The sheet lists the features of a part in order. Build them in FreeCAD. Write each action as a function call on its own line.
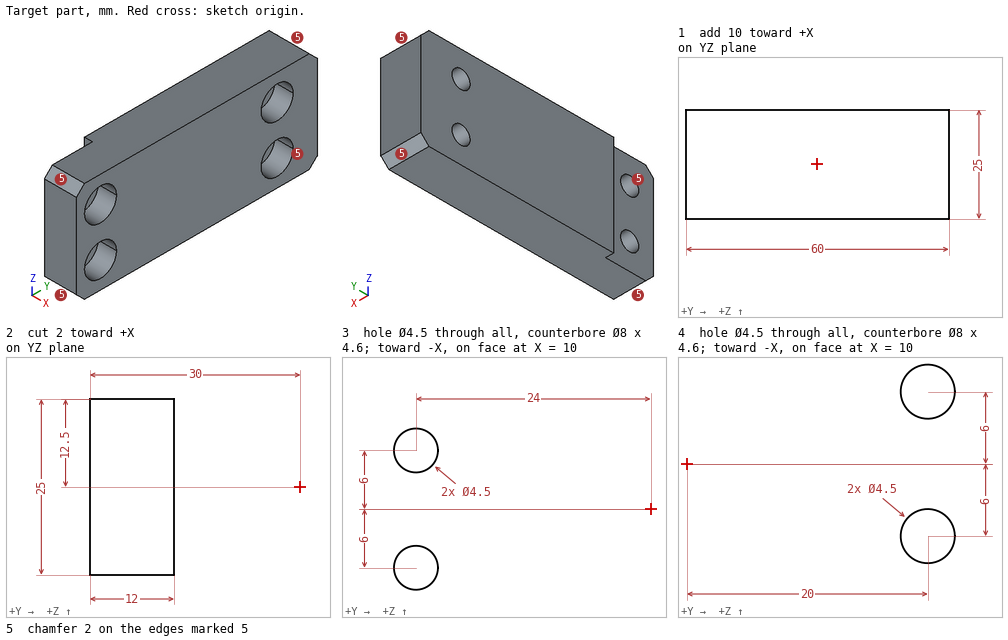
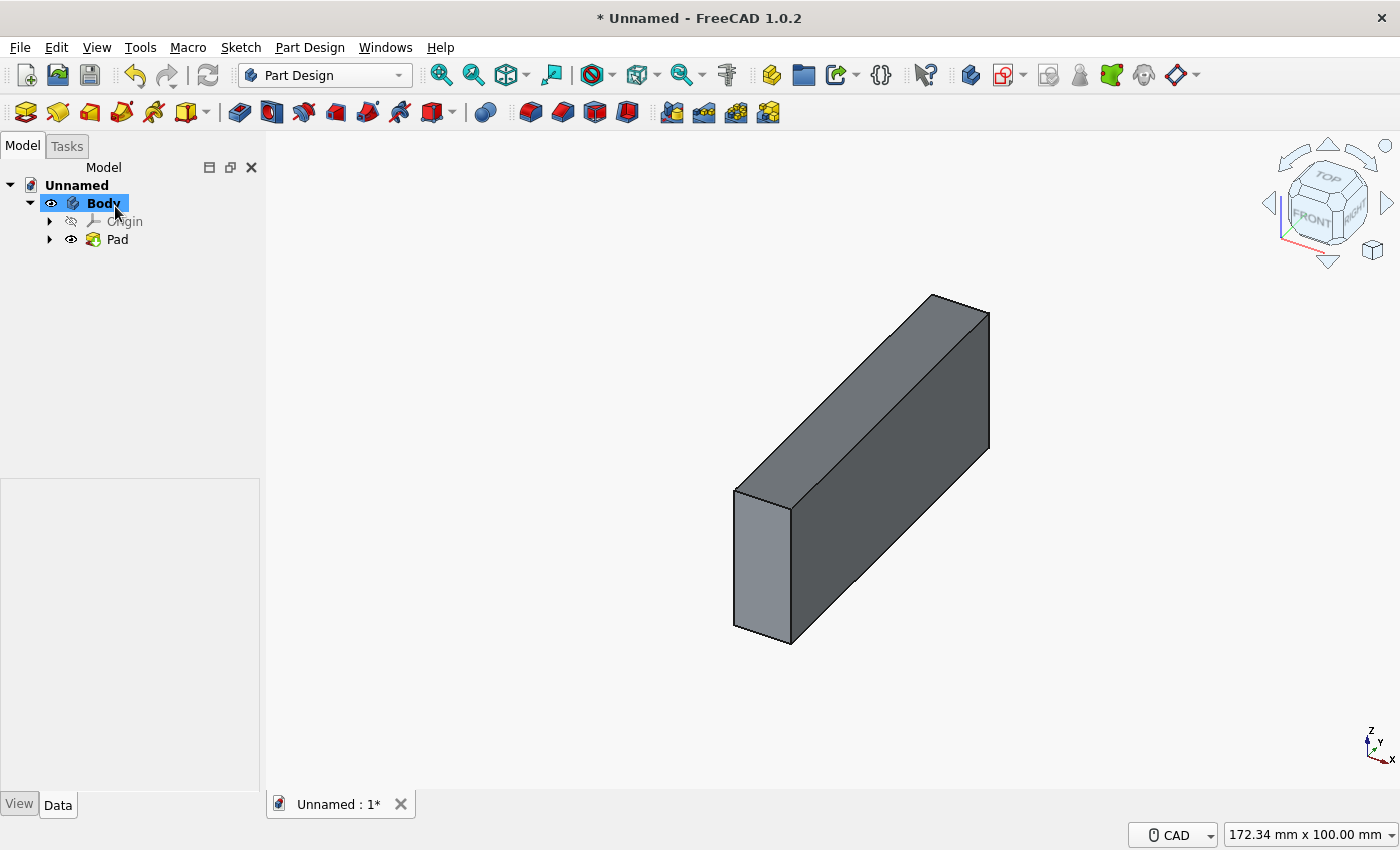
click(1004, 76)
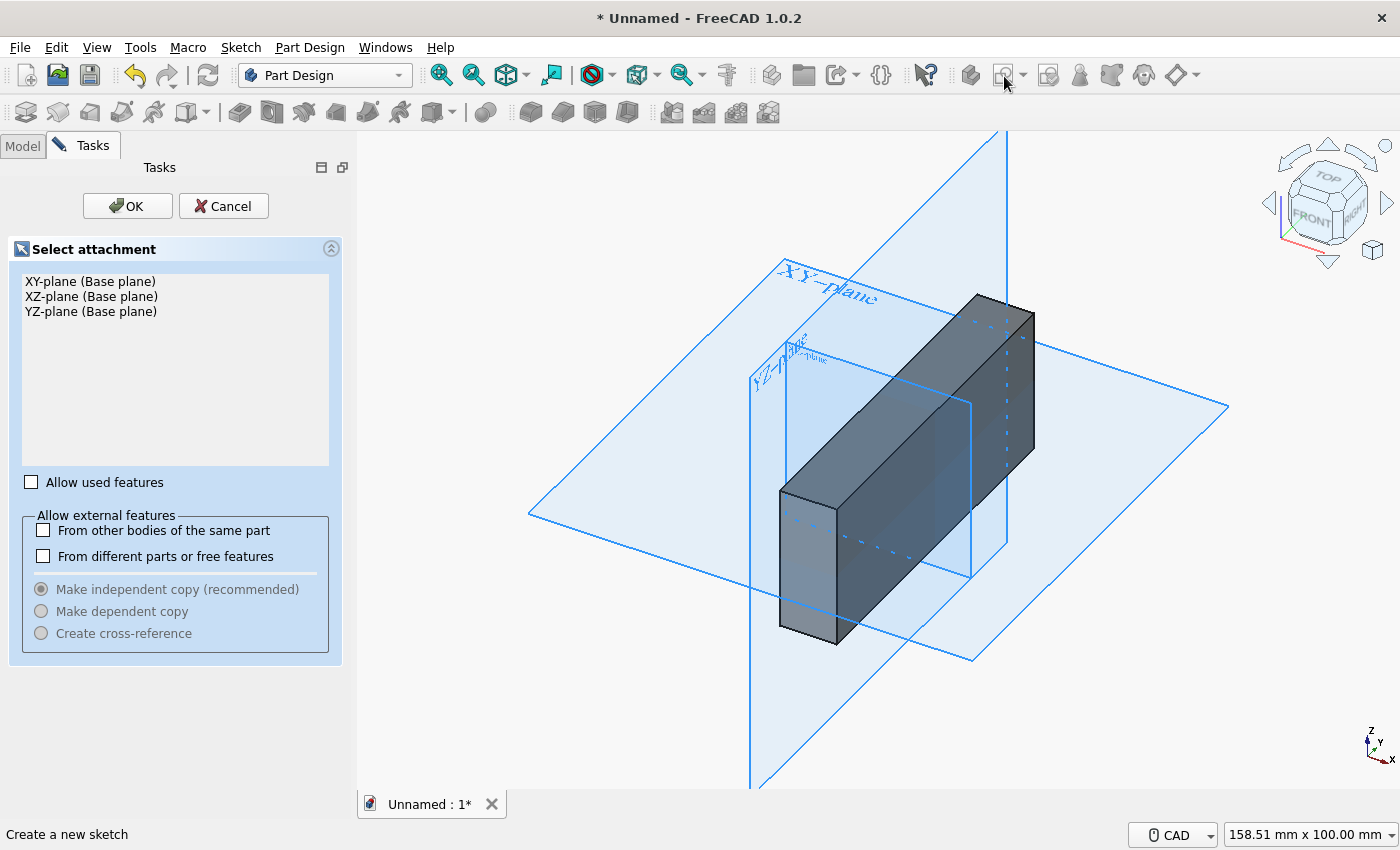
click(82, 312)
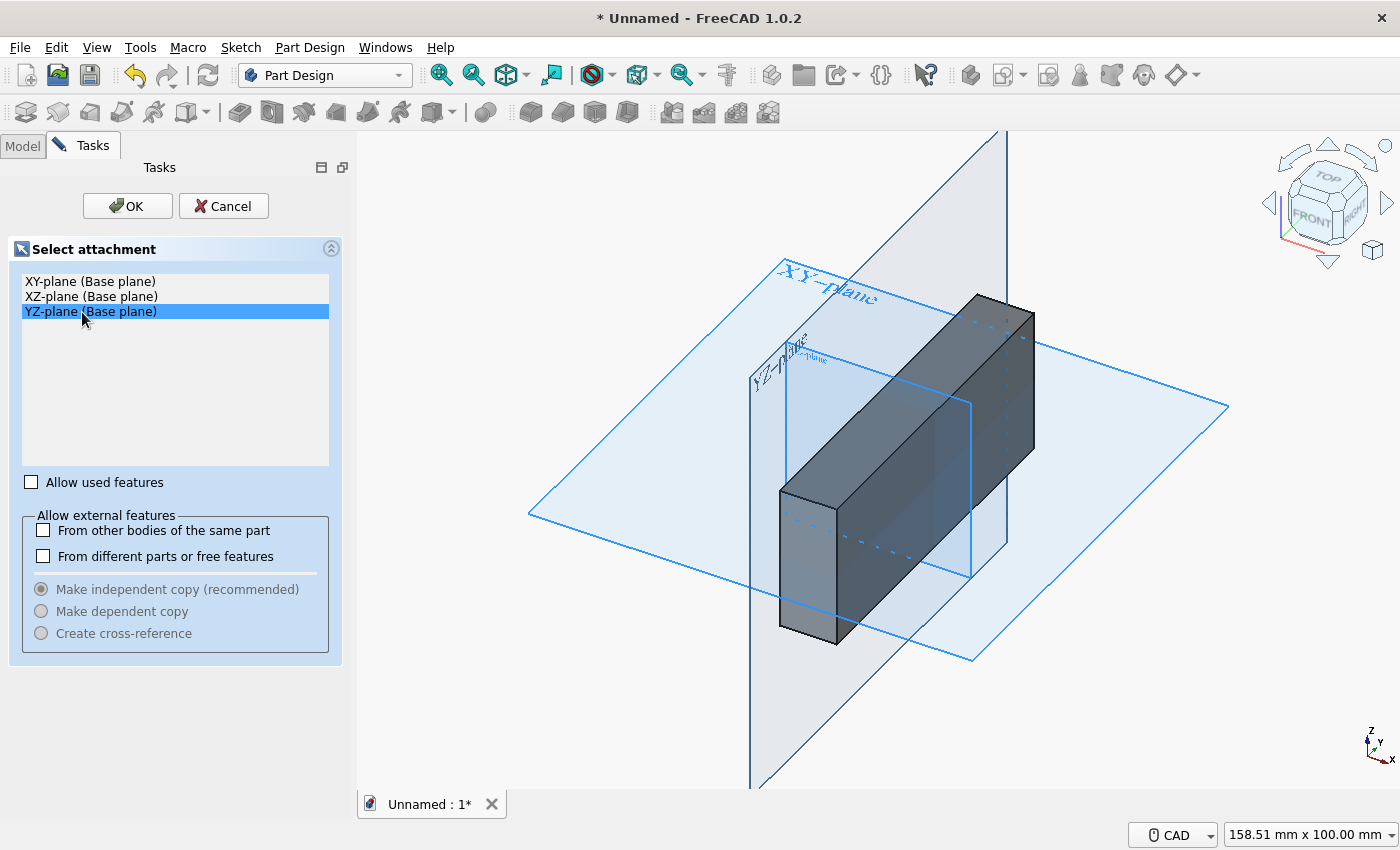
click(128, 206)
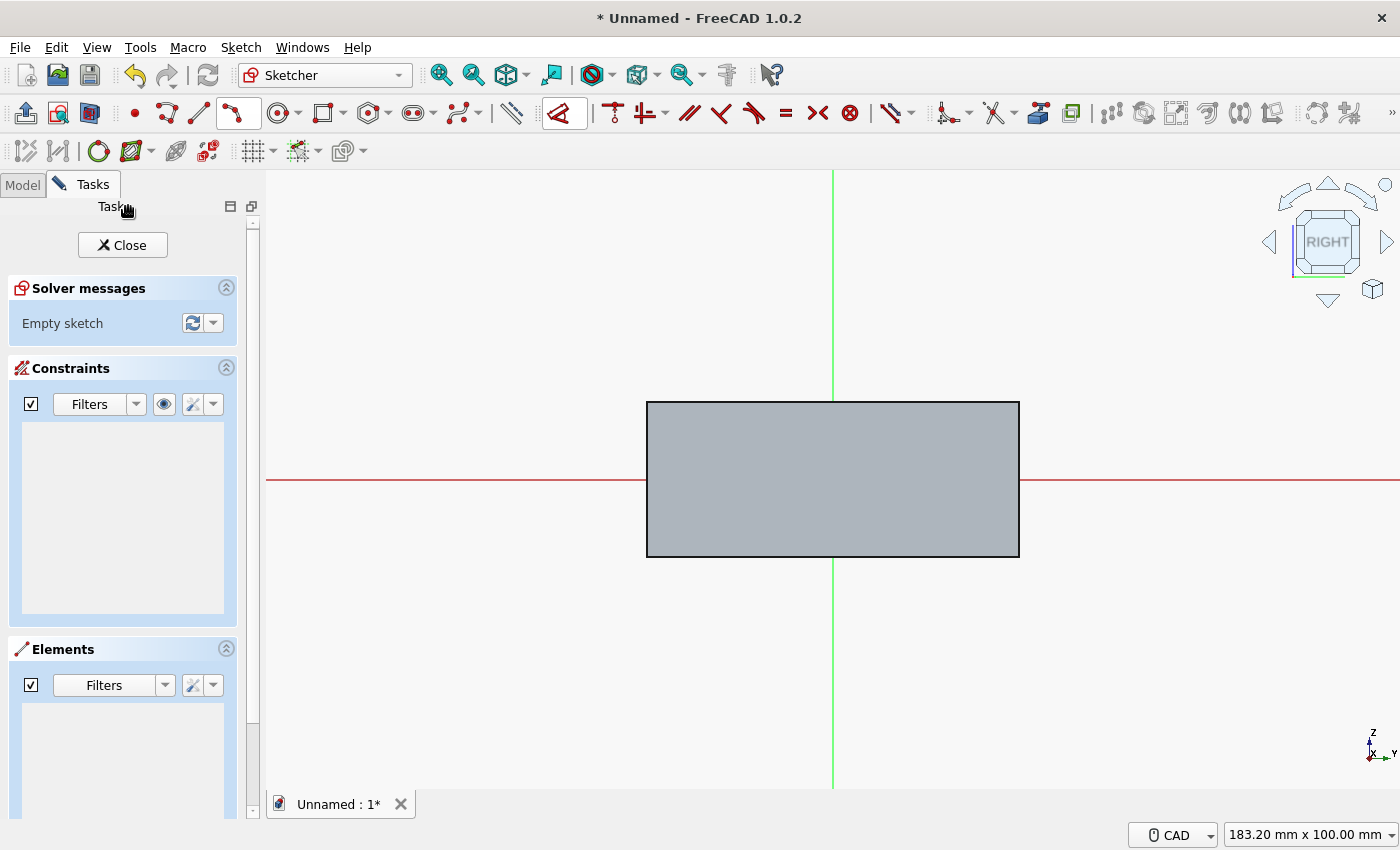
click(90, 114)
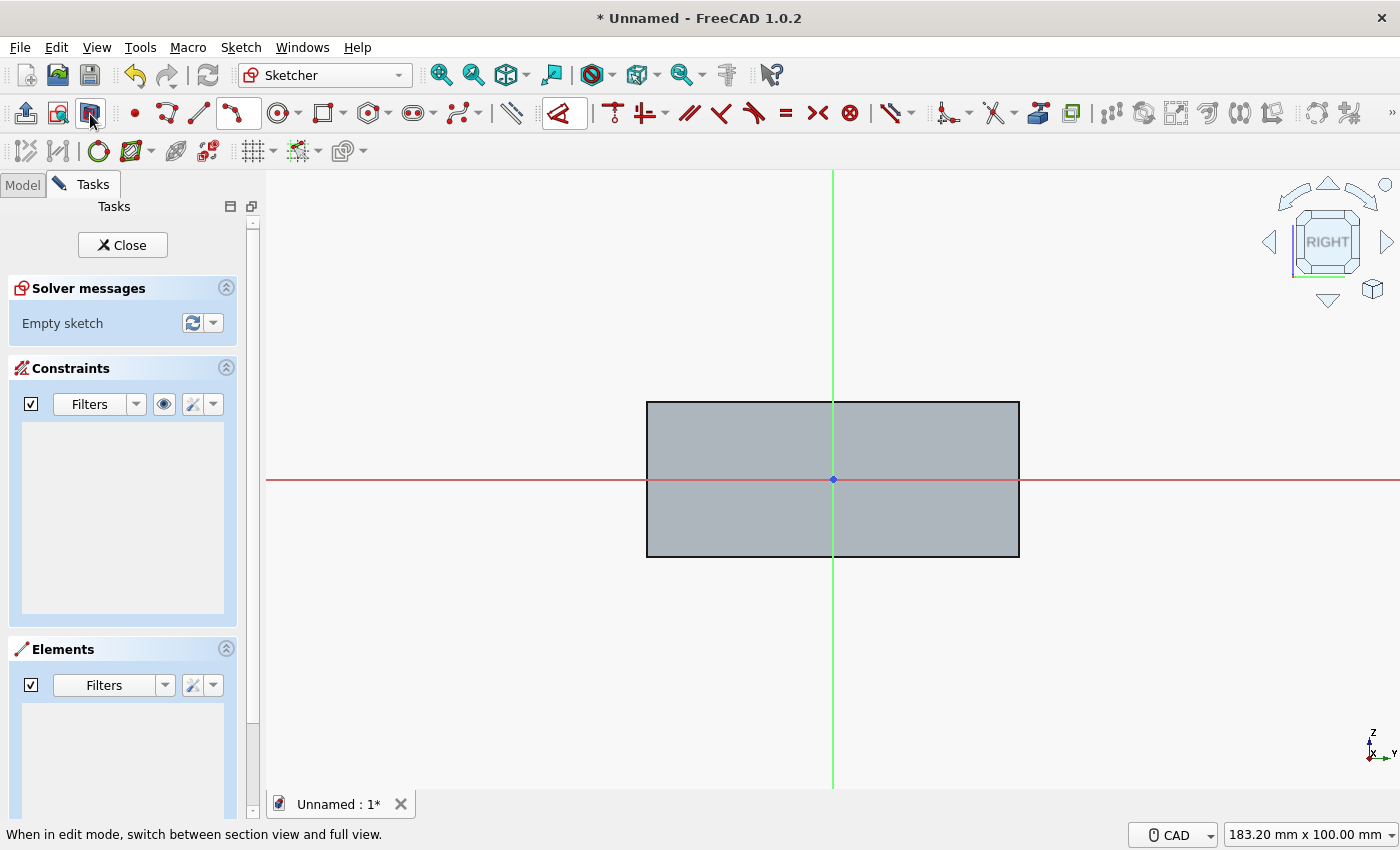
scroll(726, 480, up, 5)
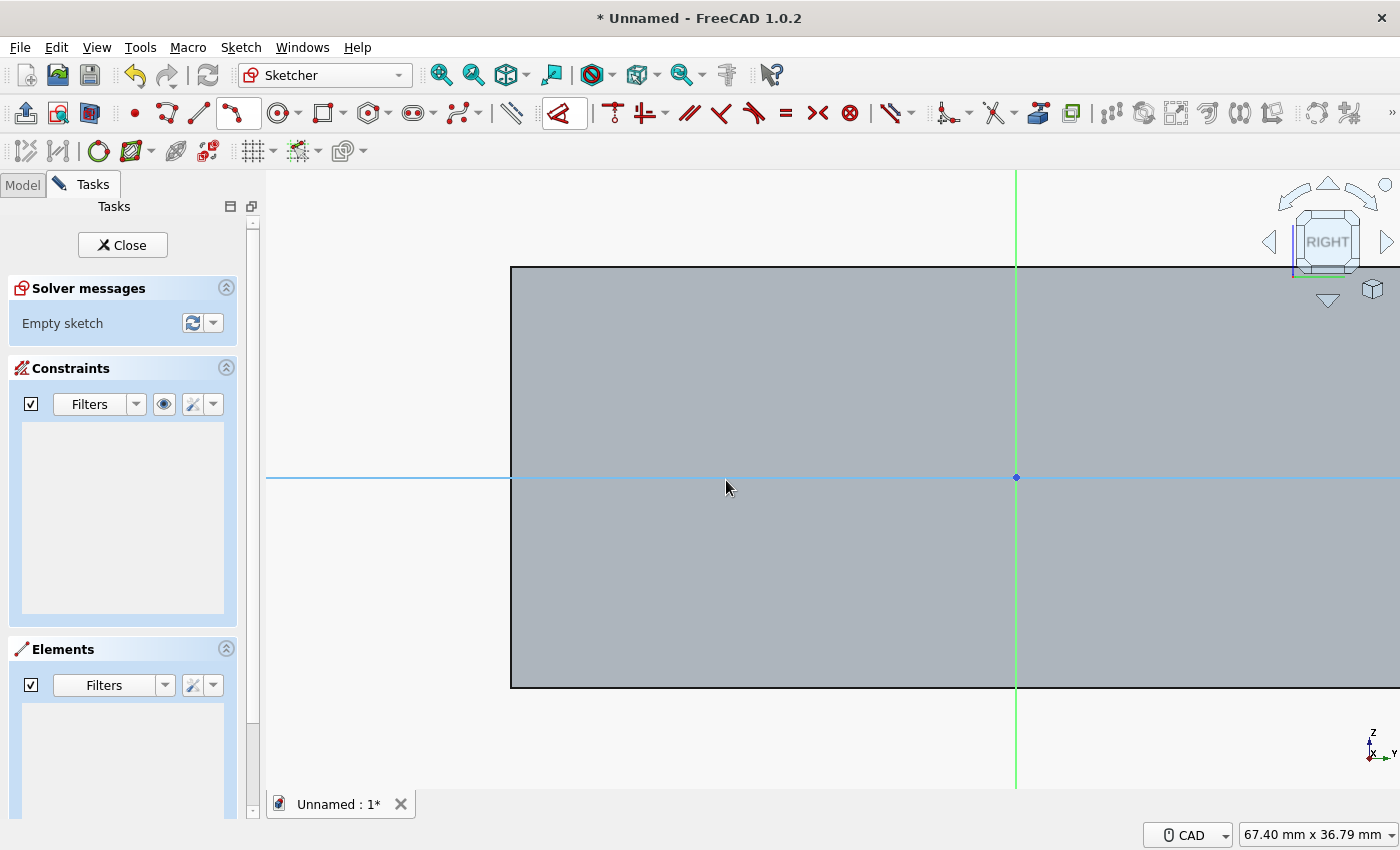
click(324, 114)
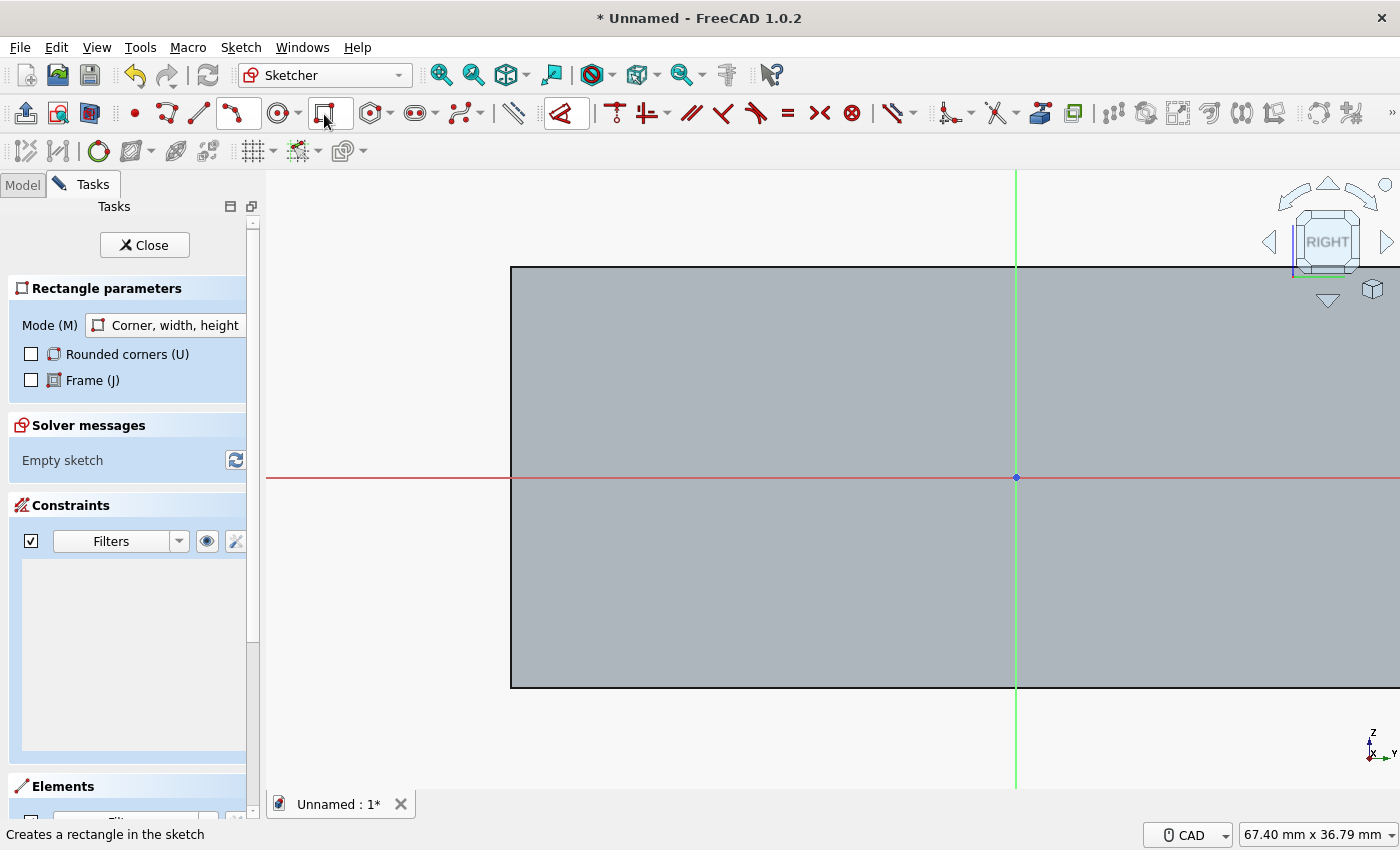
click(511, 267)
click(713, 688)
key(Escape)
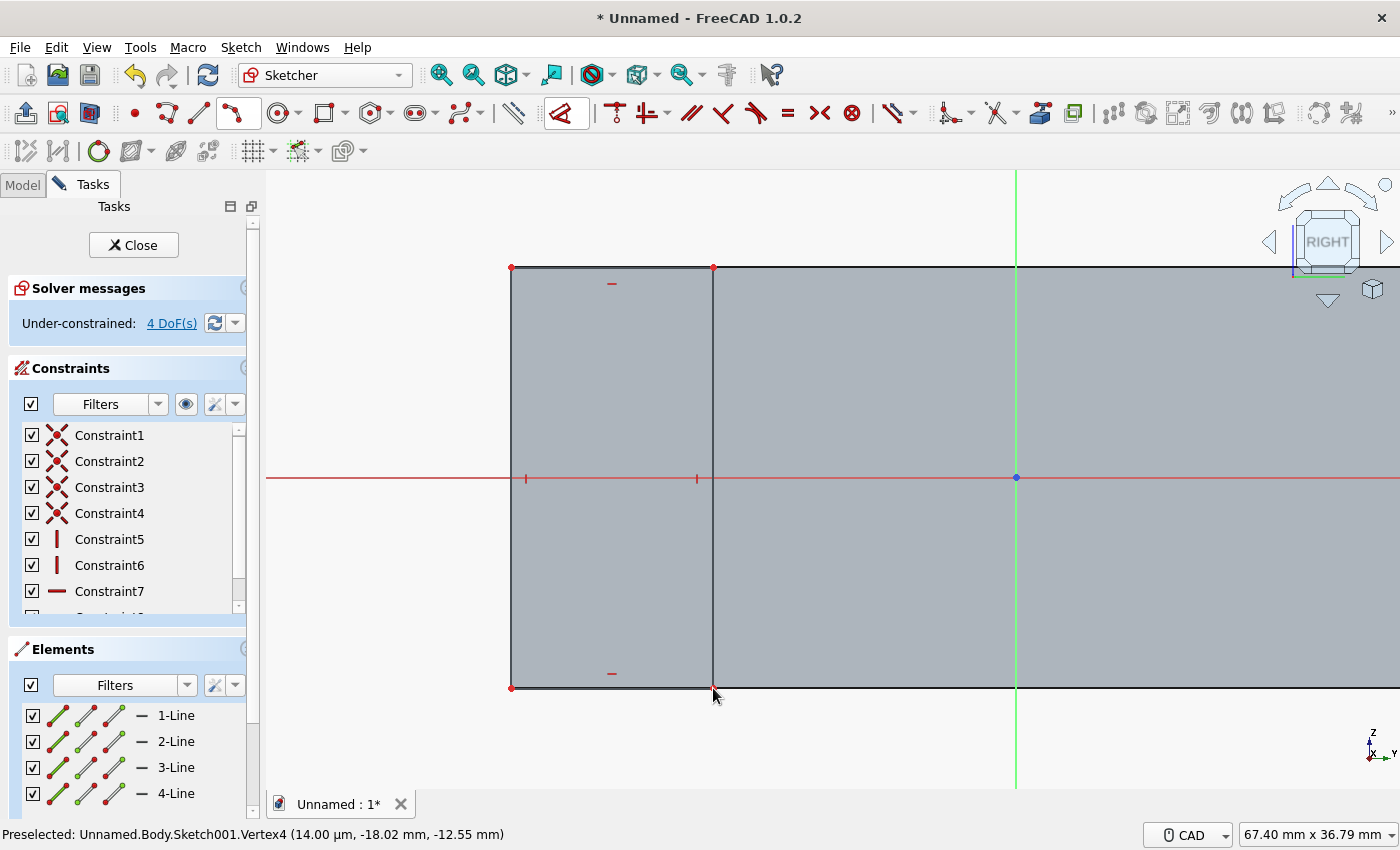
click(511, 394)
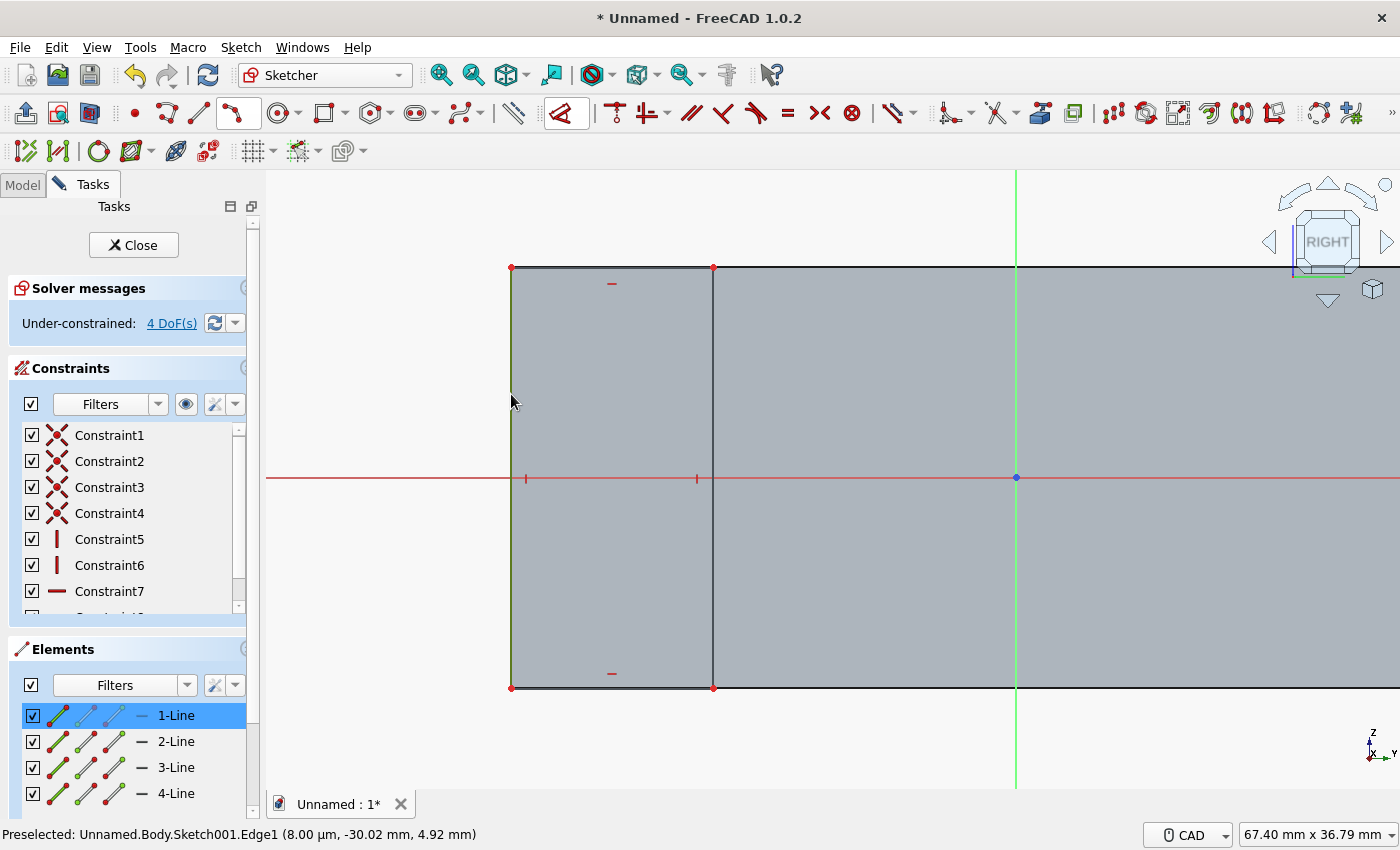
key(i)